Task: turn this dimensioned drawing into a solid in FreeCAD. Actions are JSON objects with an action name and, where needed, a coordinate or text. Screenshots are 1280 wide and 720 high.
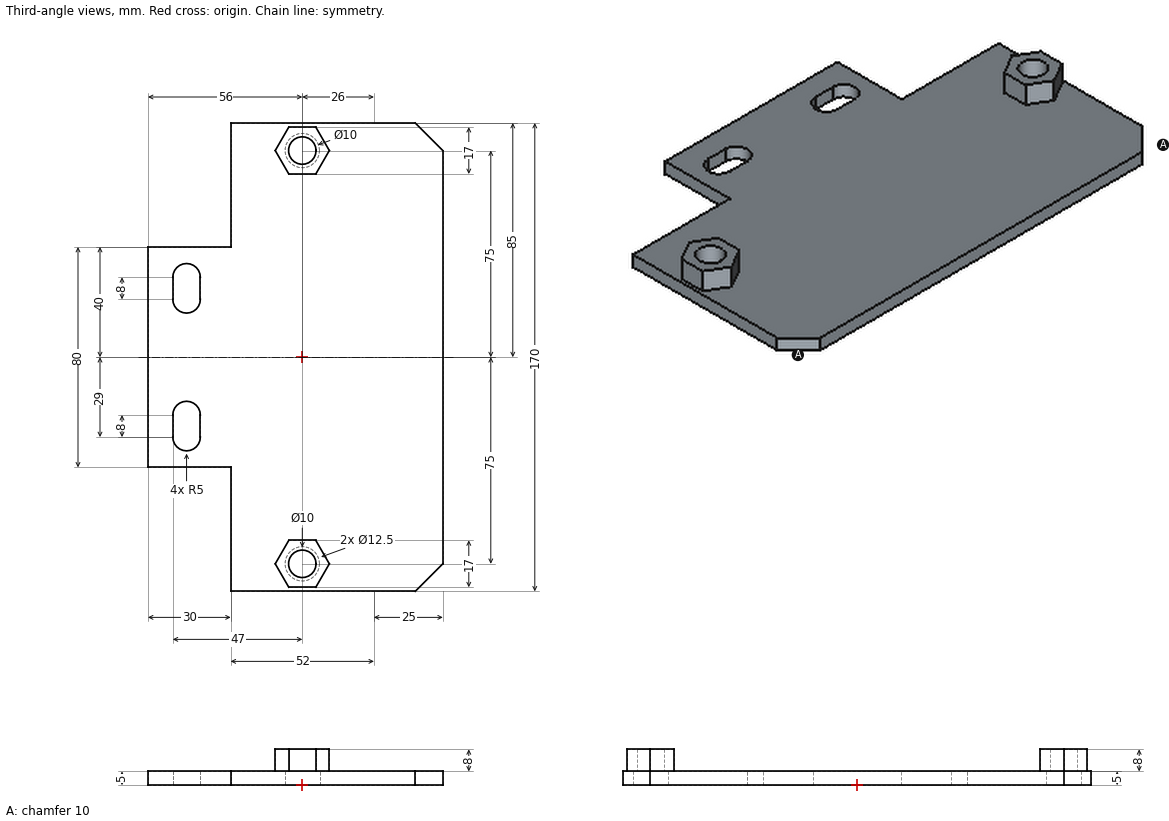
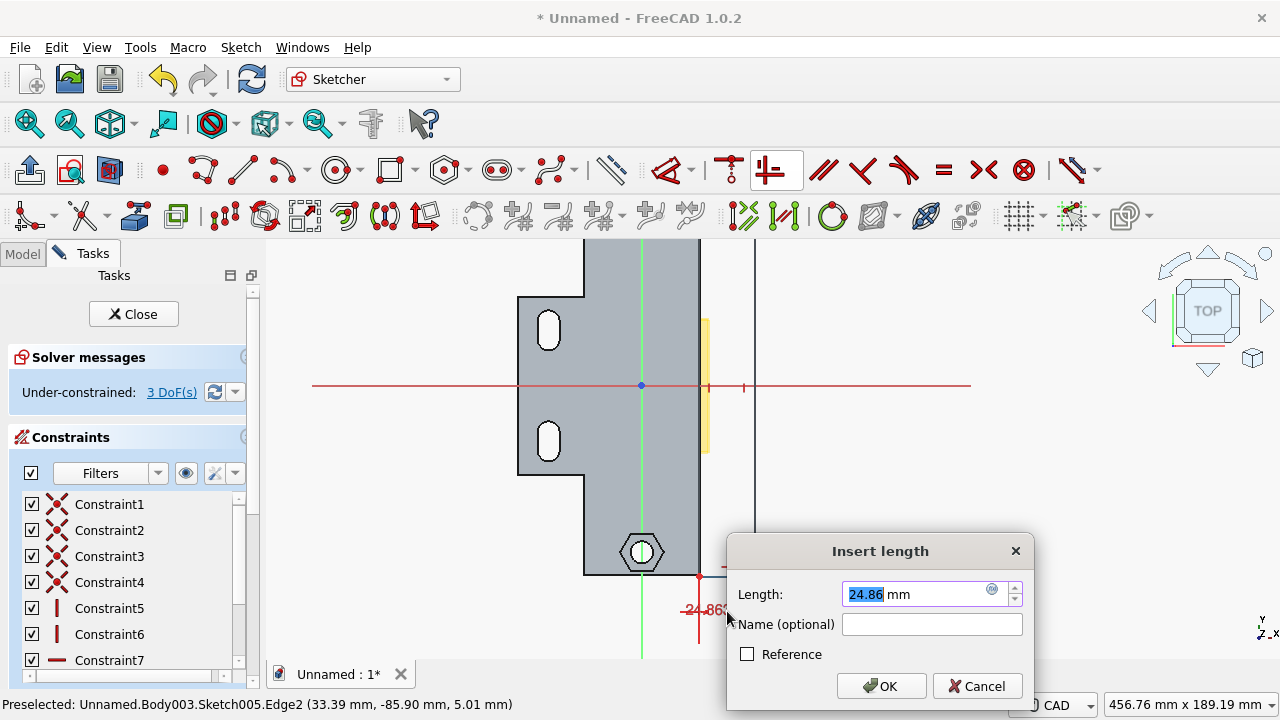
{"action": "type", "text": "25"}
{"action": "key", "text": "Return"}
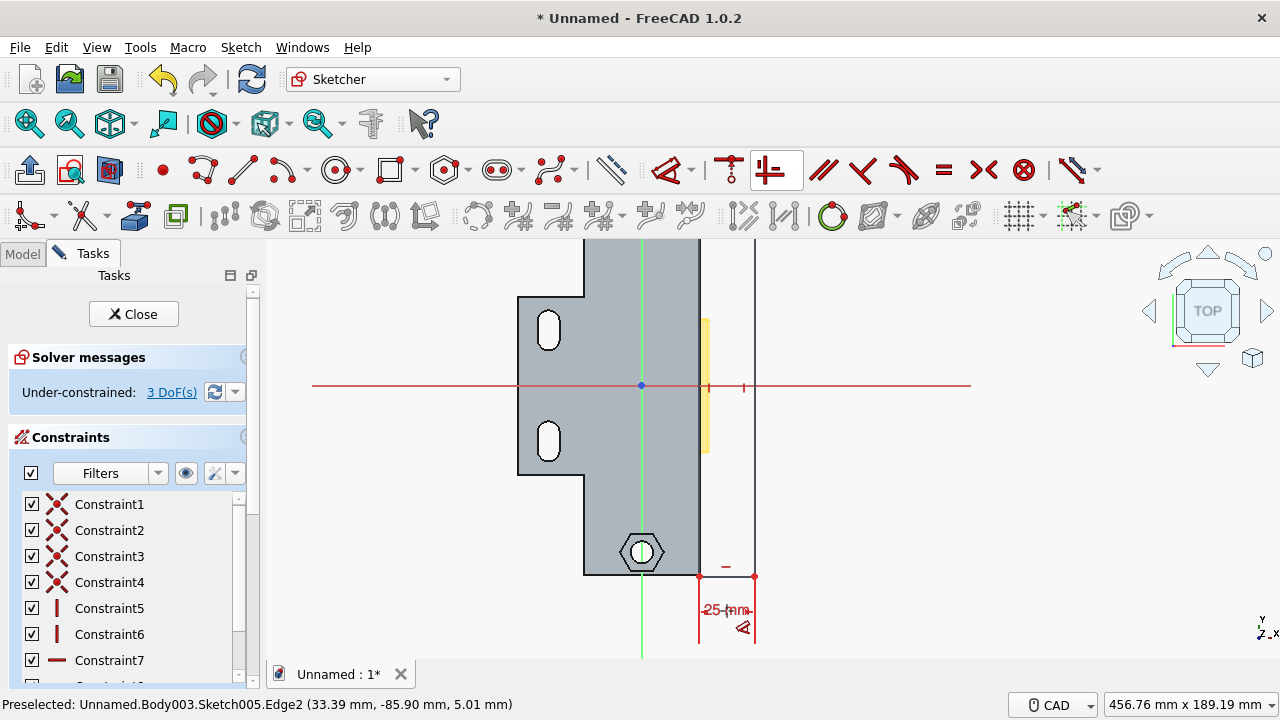
{"action": "left_click", "coordinate": [699, 312]}
{"action": "left_click", "coordinate": [733, 422]}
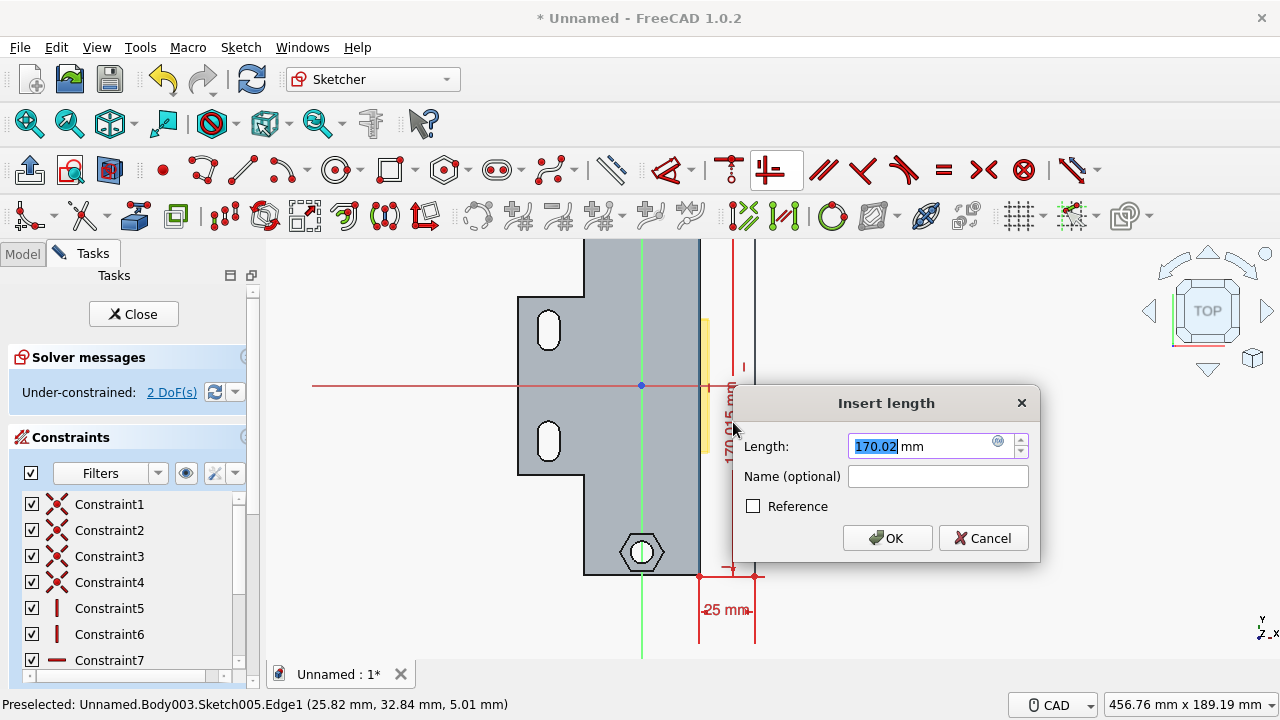
{"action": "type", "text": "170"}
{"action": "key", "text": "Return"}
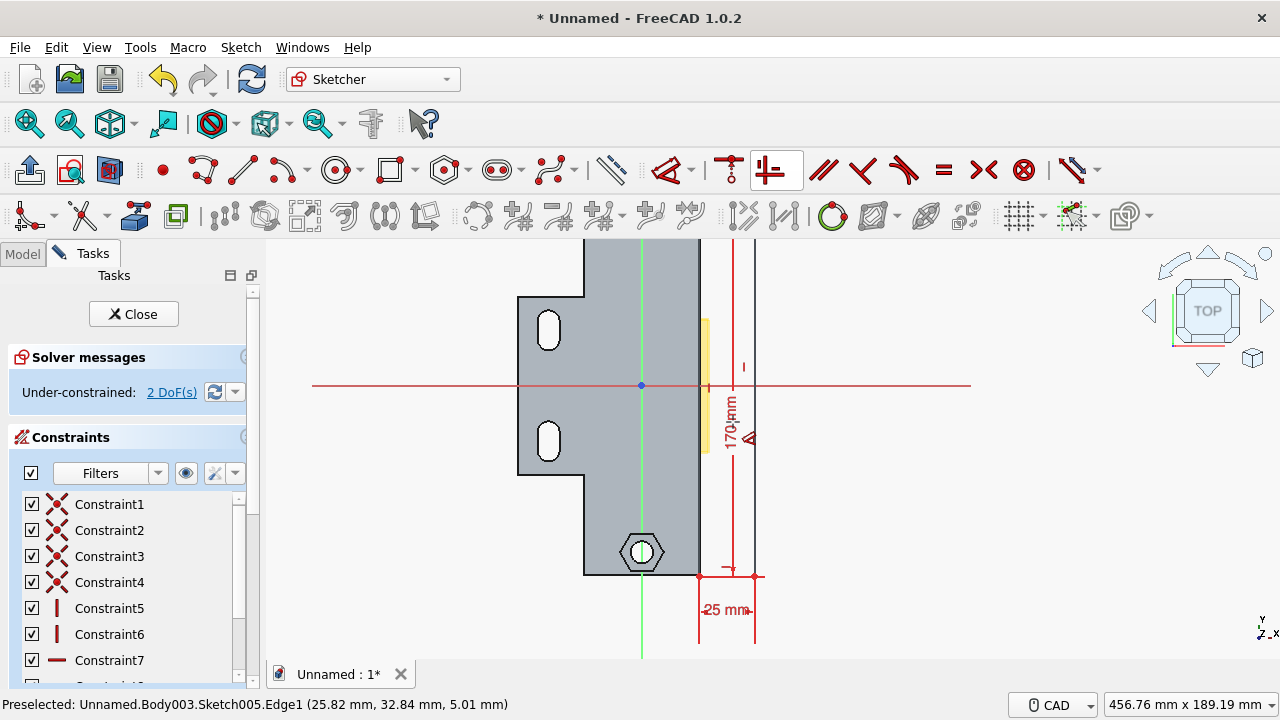
{"action": "scroll", "coordinate": [717, 577], "scroll_direction": "down", "scroll_amount": 2}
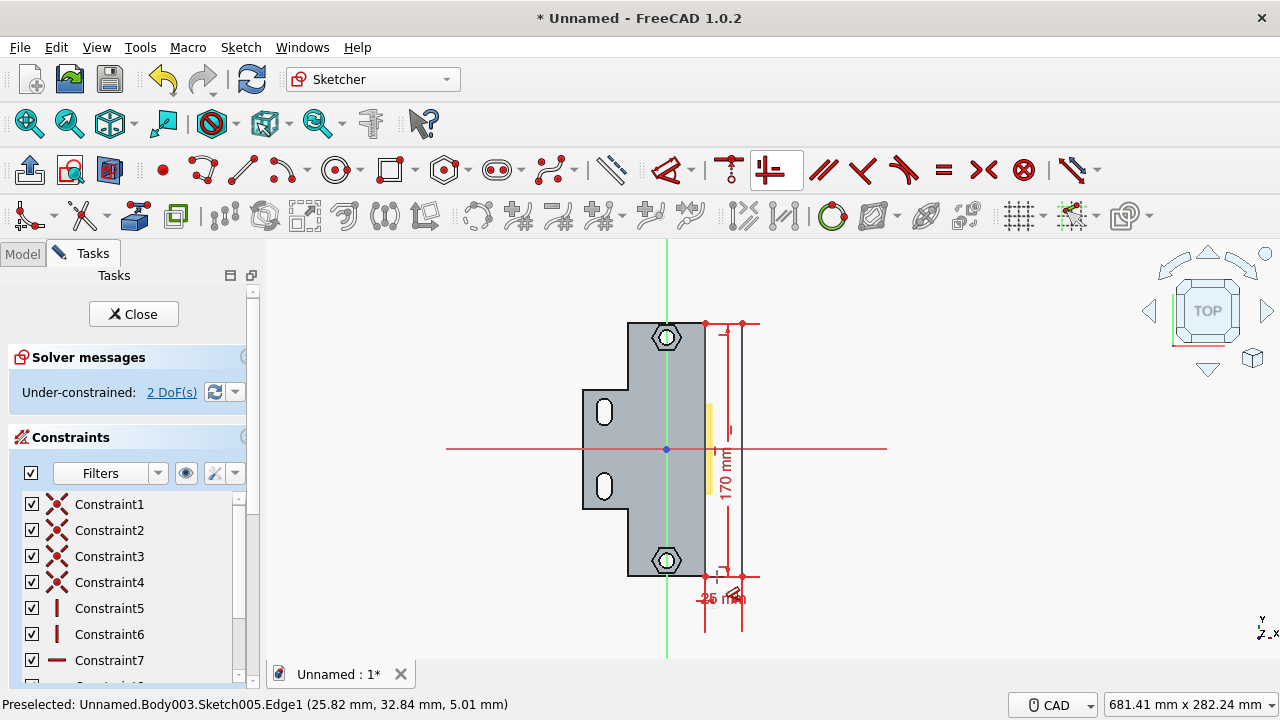
{"action": "left_click", "coordinate": [705, 324]}
{"action": "left_click", "coordinate": [686, 290]}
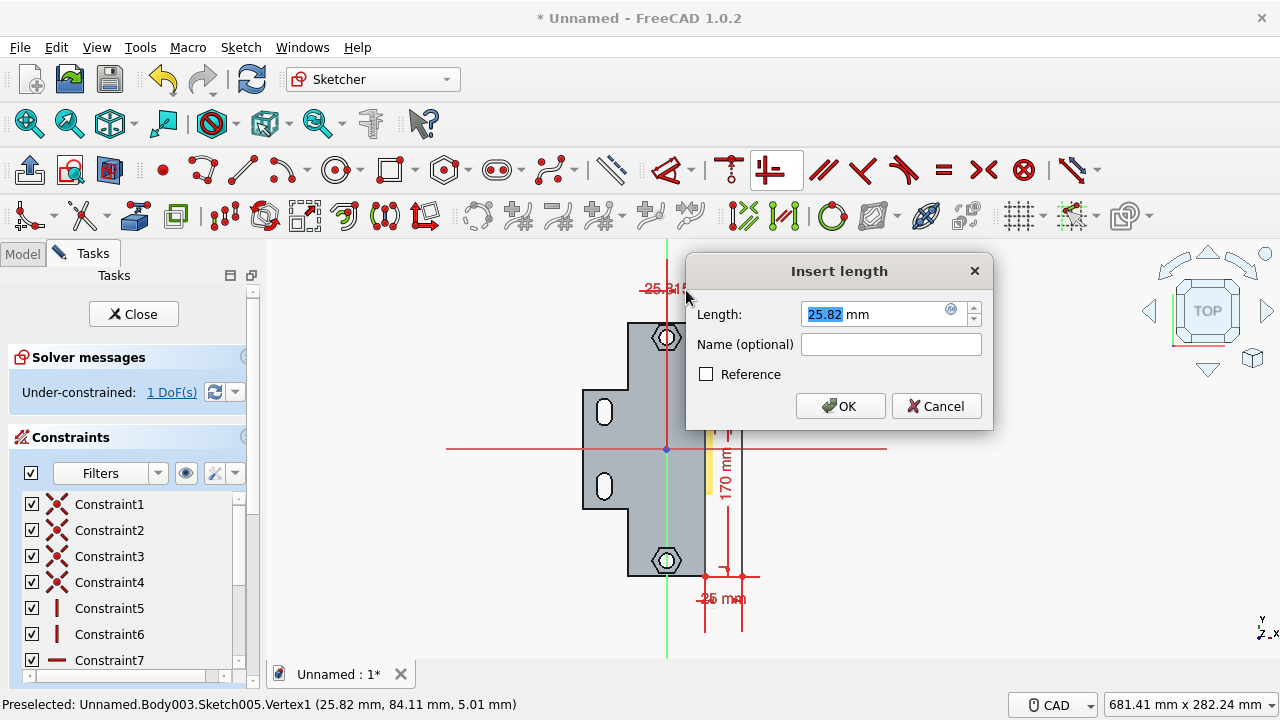
{"action": "type", "text": "26"}
{"action": "key", "text": "Return"}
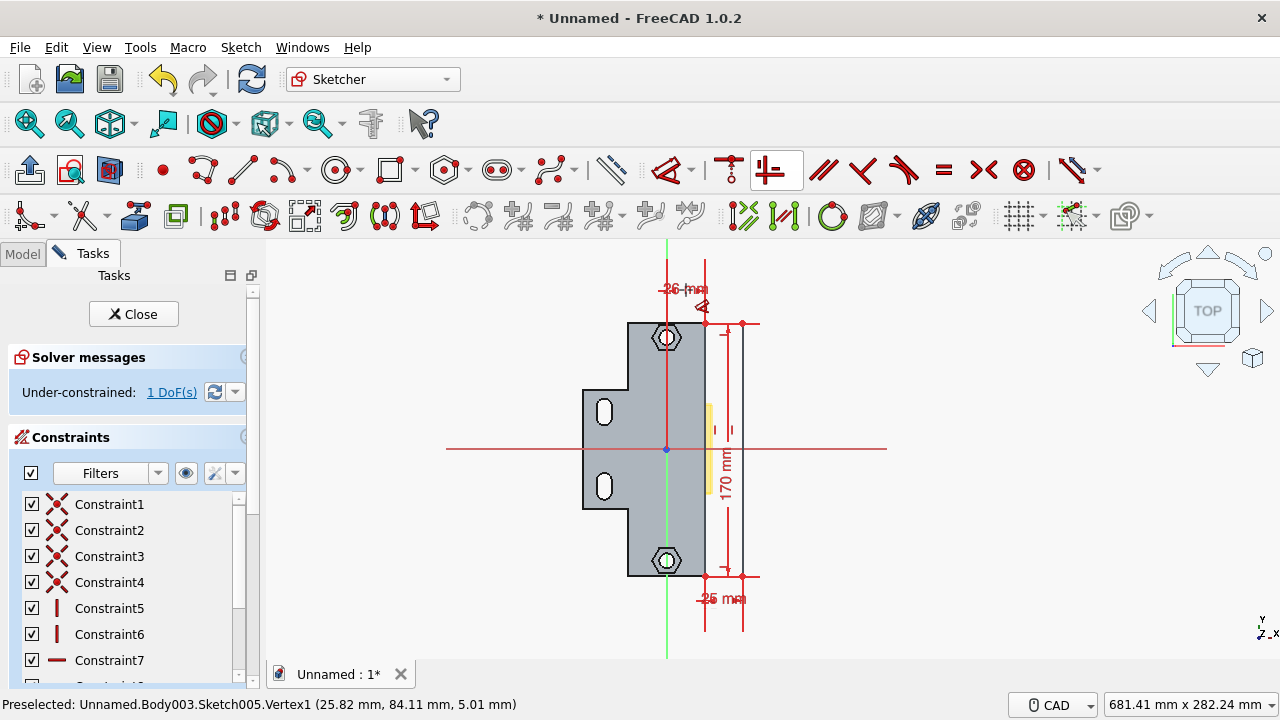
{"action": "left_click", "coordinate": [705, 324]}
{"action": "left_click", "coordinate": [633, 387]}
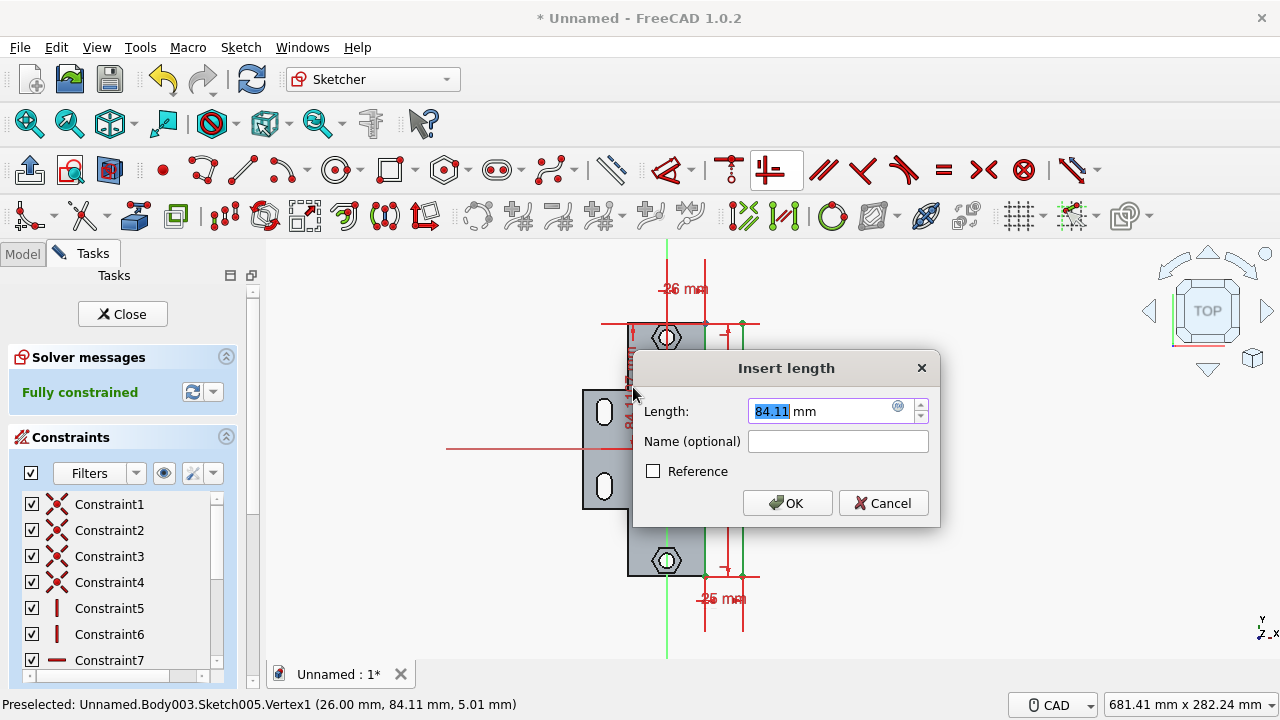
{"action": "type", "text": "85"}
{"action": "key", "text": "Return"}
{"action": "key", "text": "Escape"}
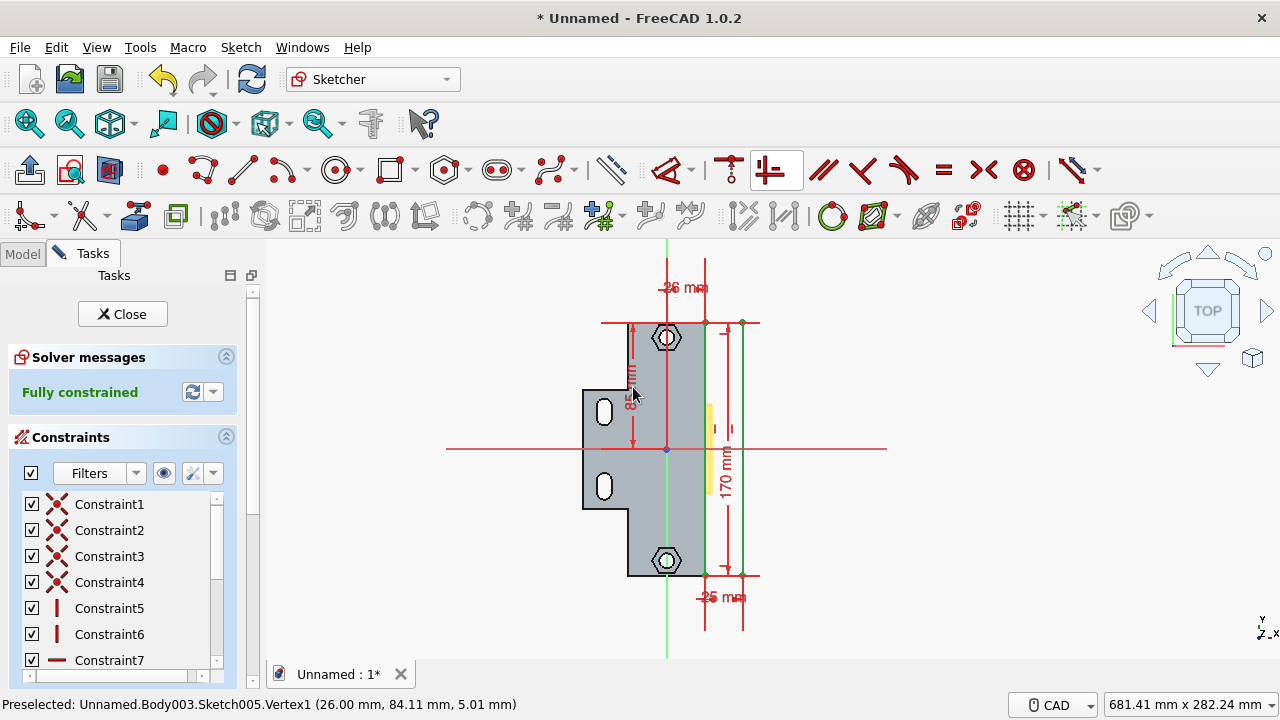
{"action": "left_click", "coordinate": [123, 314]}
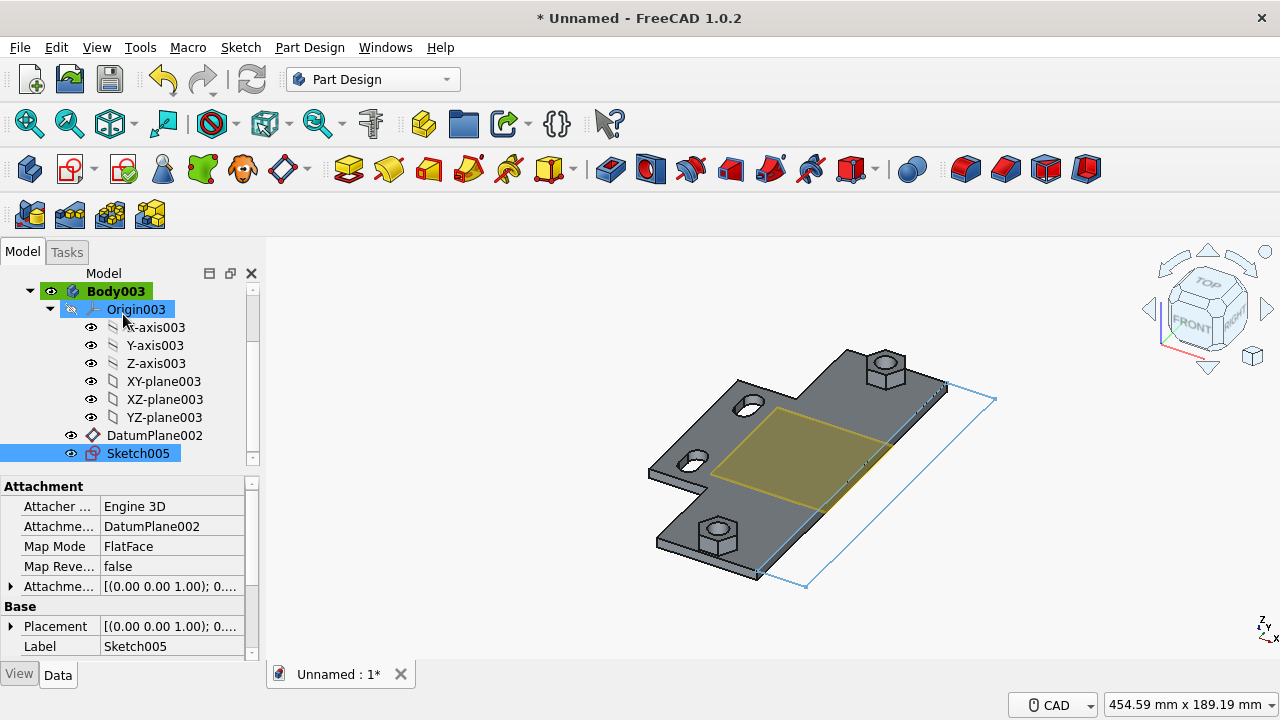
{"action": "left_click", "coordinate": [350, 170]}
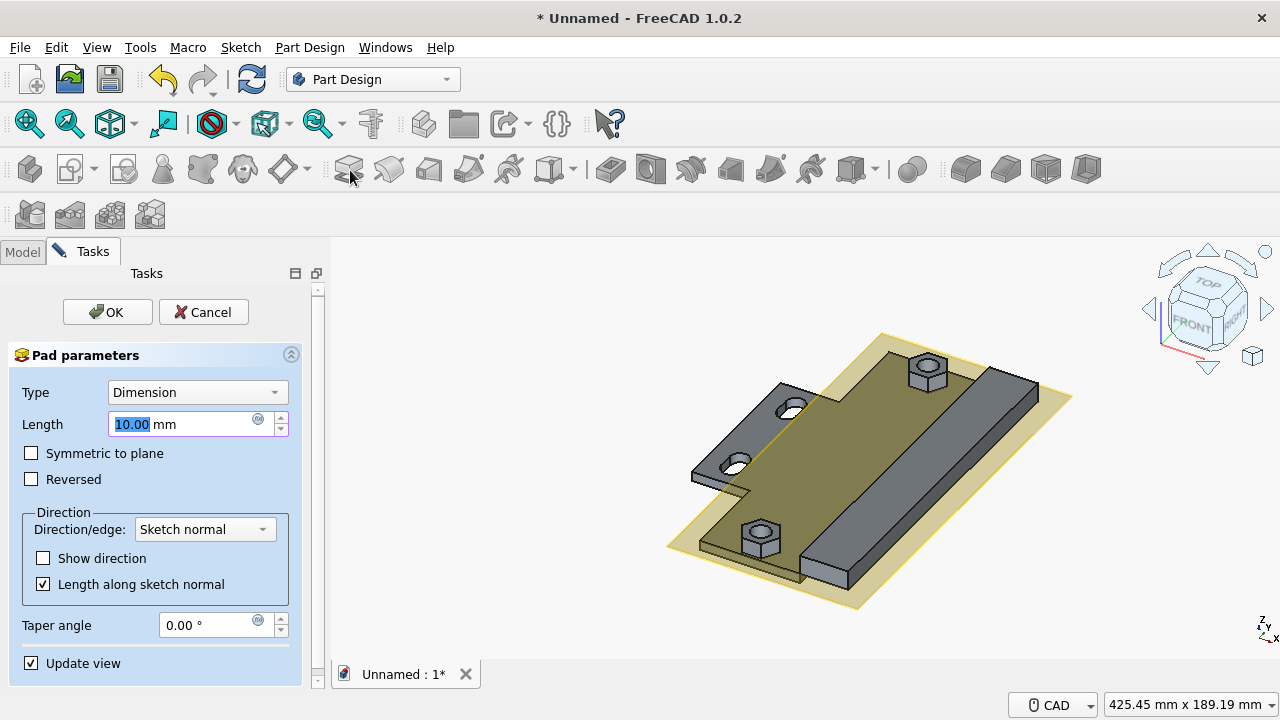
{"action": "type", "text": "5"}
{"action": "key", "text": "Tab"}